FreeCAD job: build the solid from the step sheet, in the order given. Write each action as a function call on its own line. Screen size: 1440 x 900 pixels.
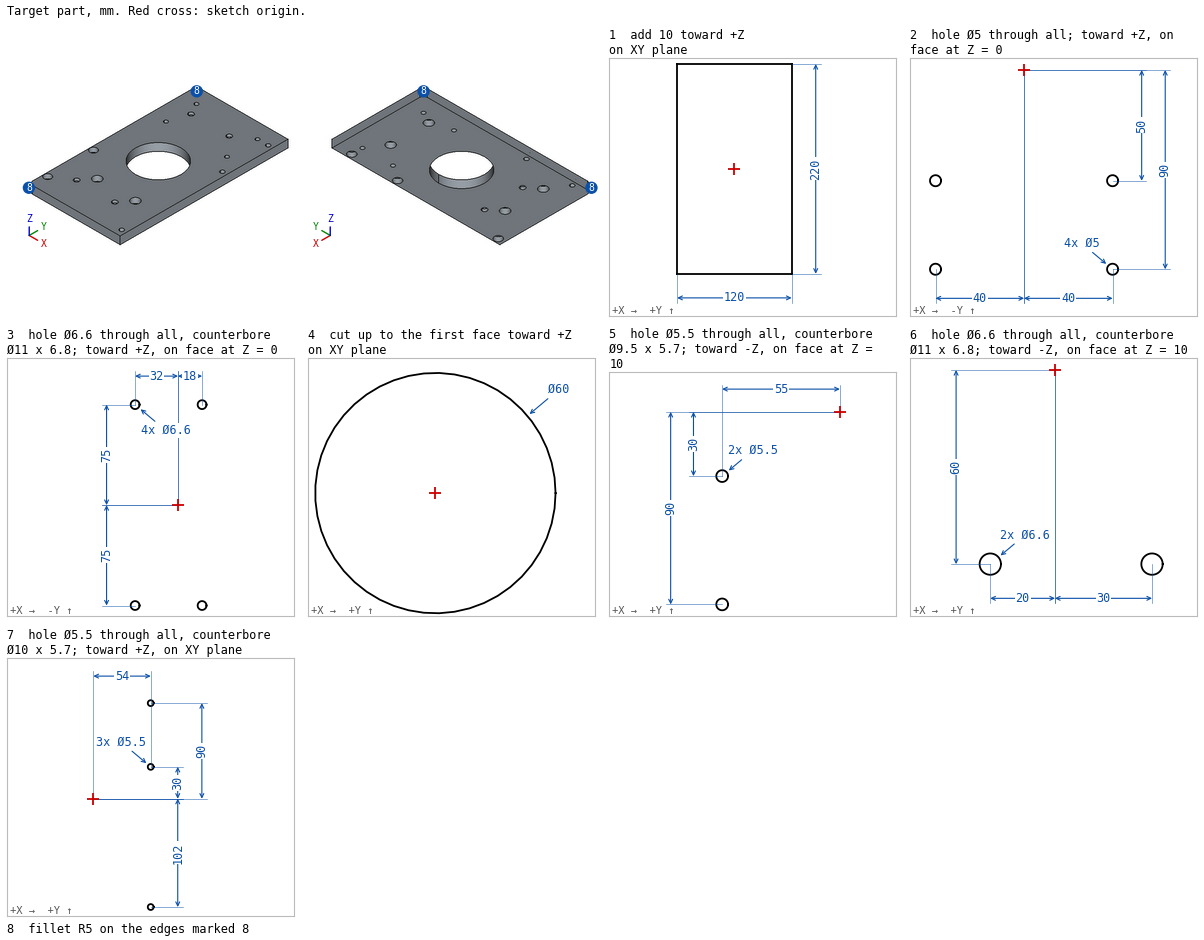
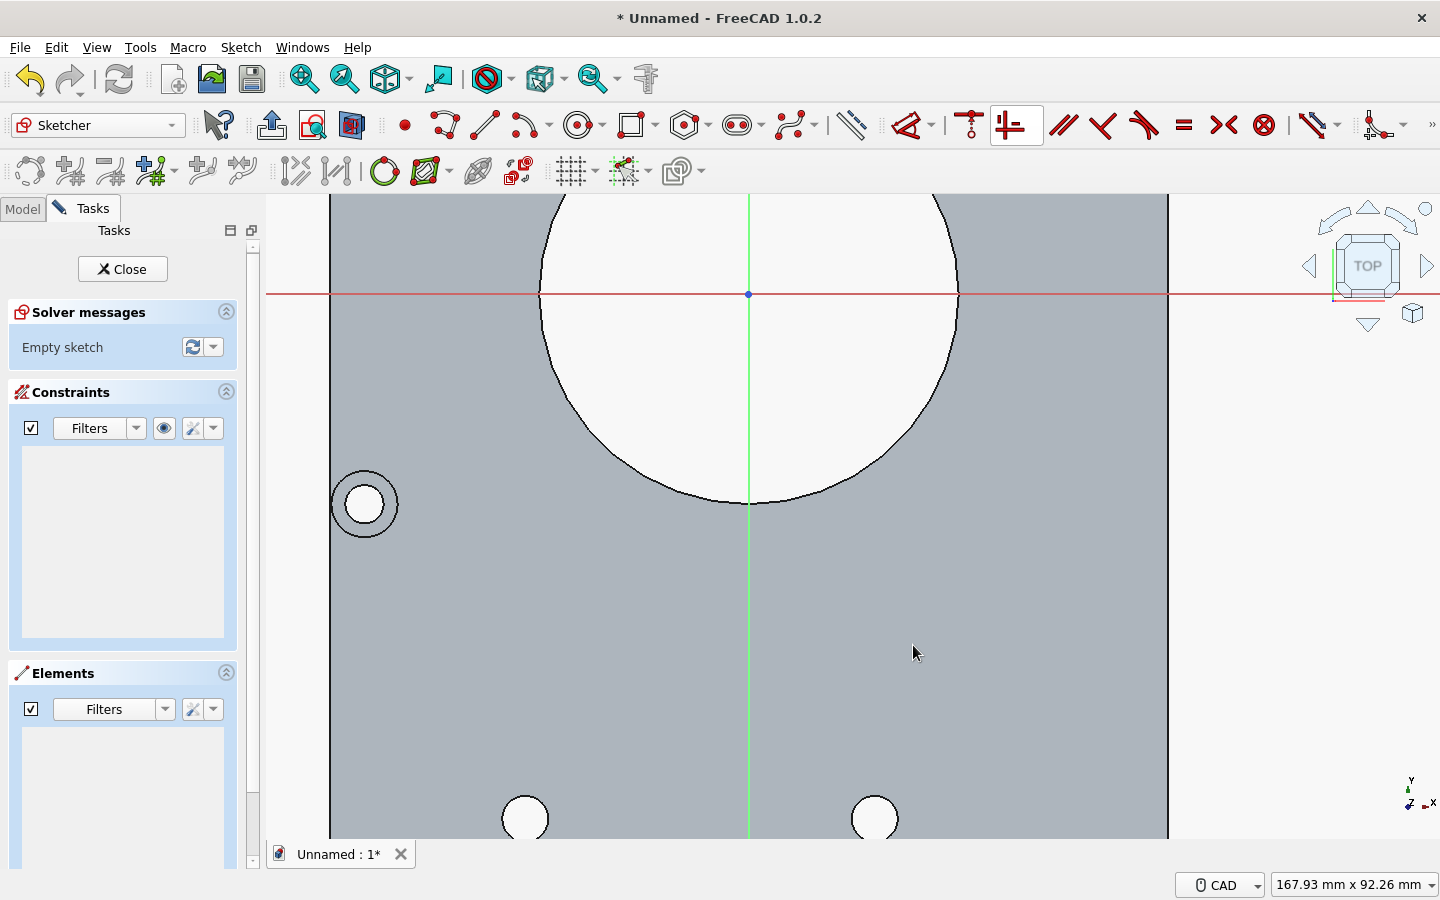
key(g)
key(c)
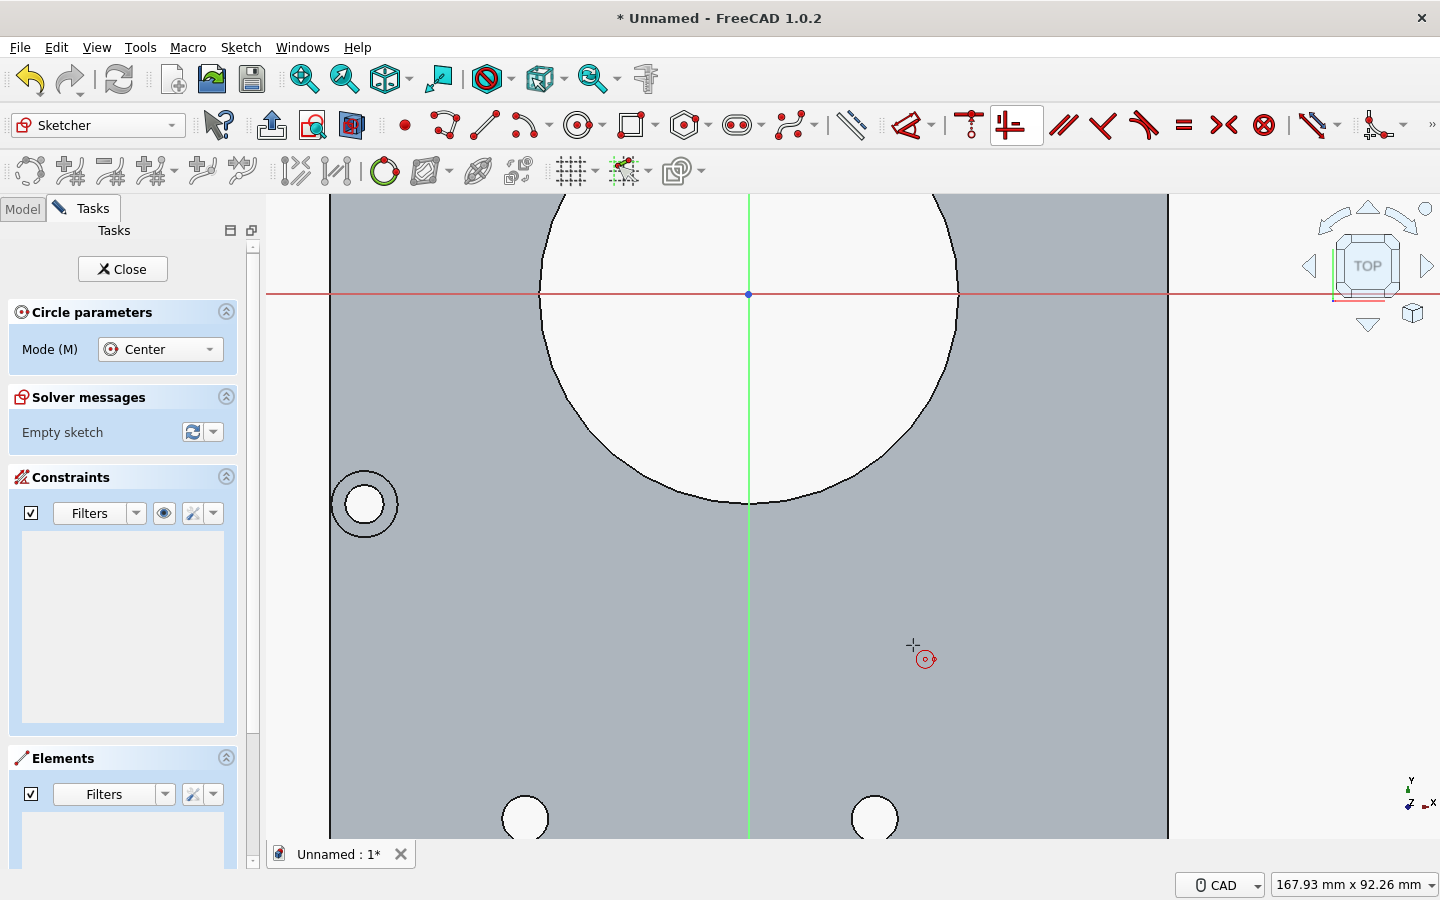
click(609, 714)
move(625, 698)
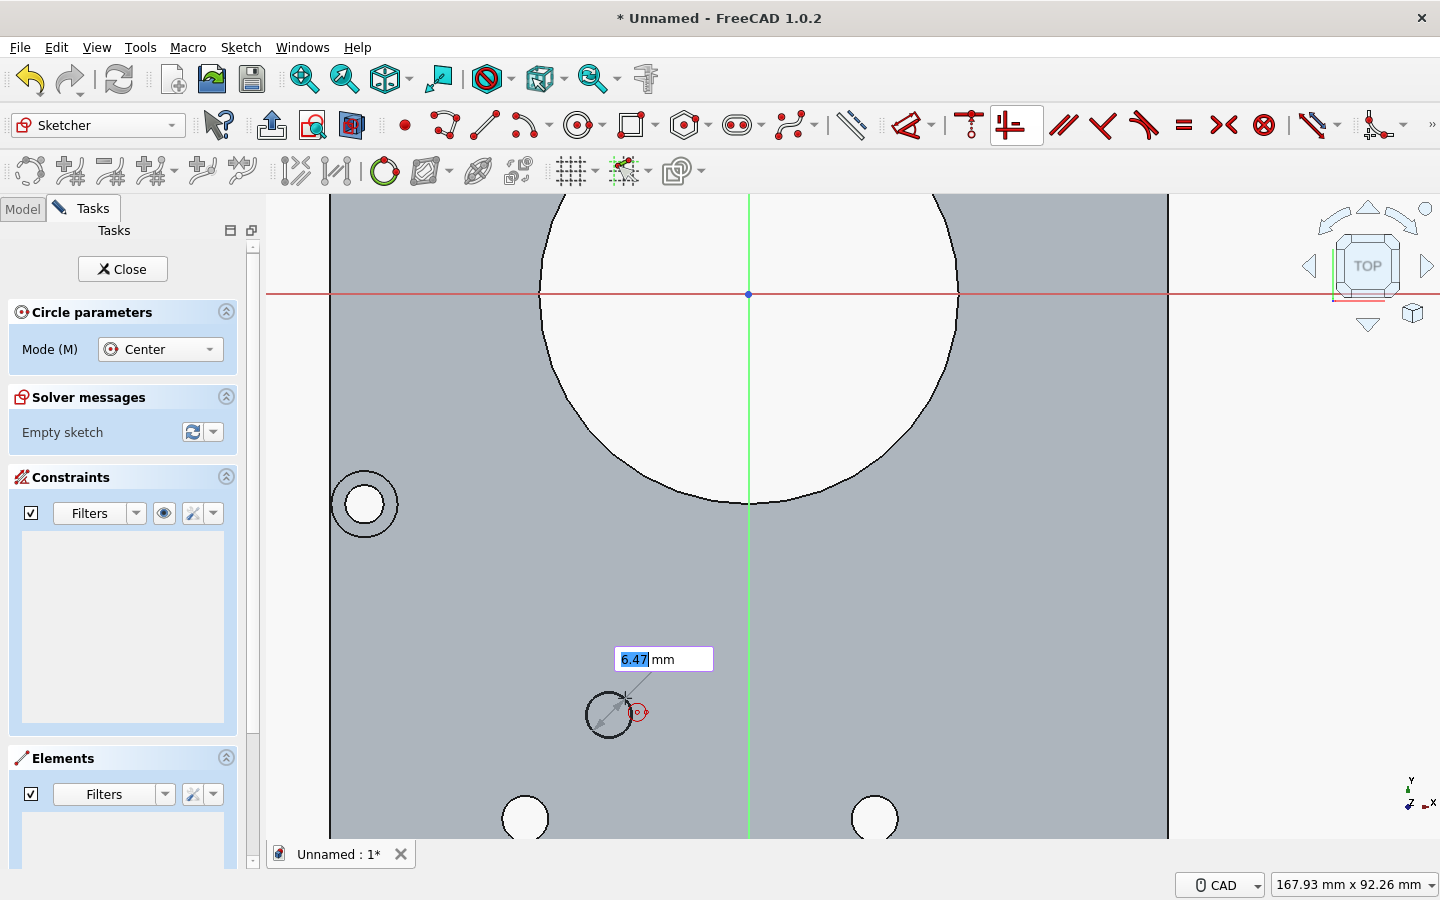
text(6.6)
key(Return)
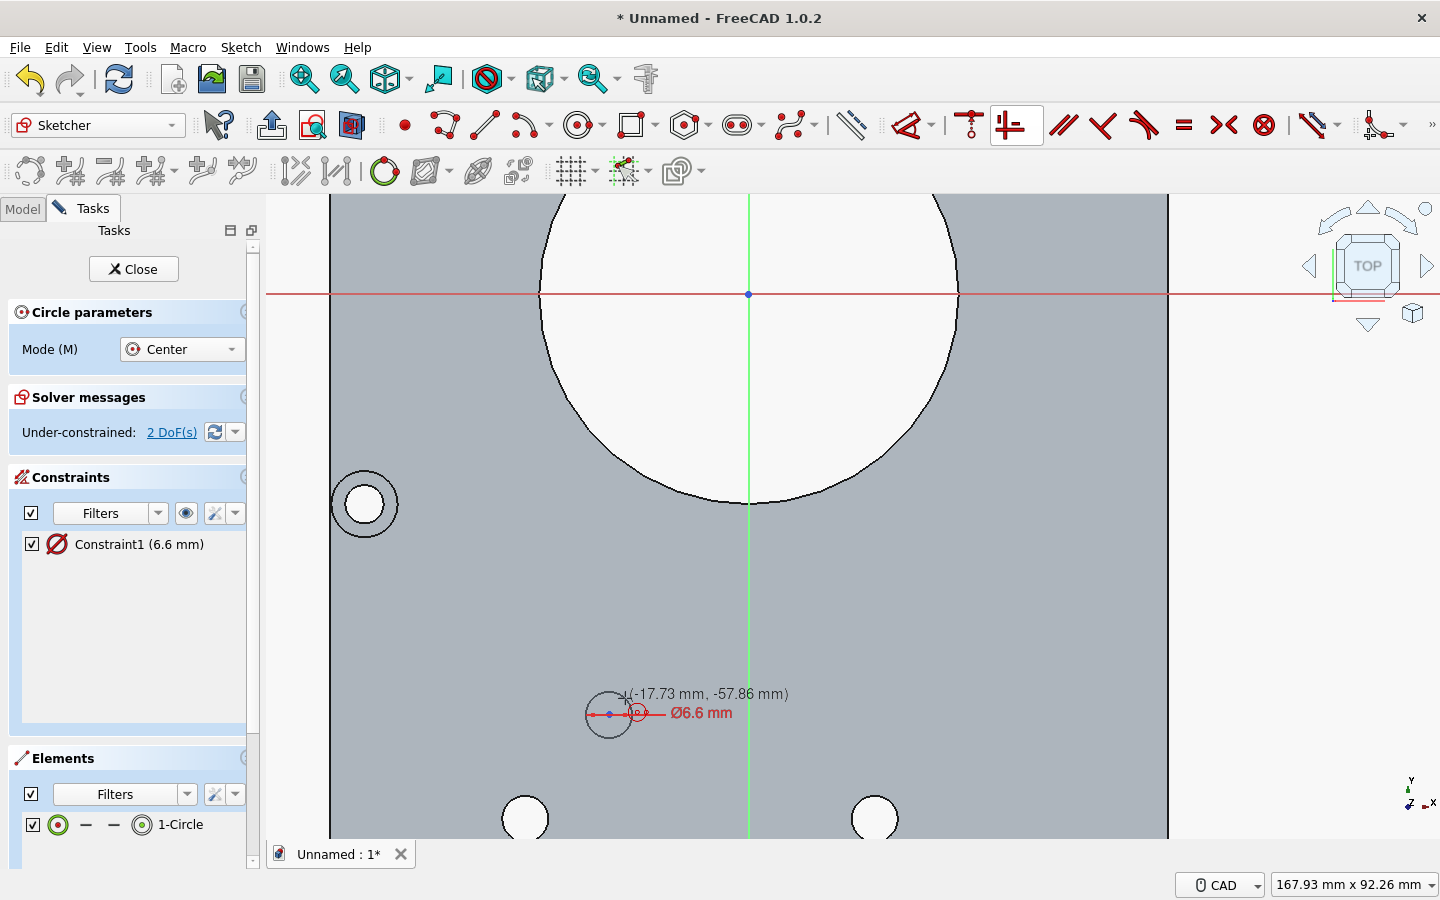
click(959, 714)
move(975, 698)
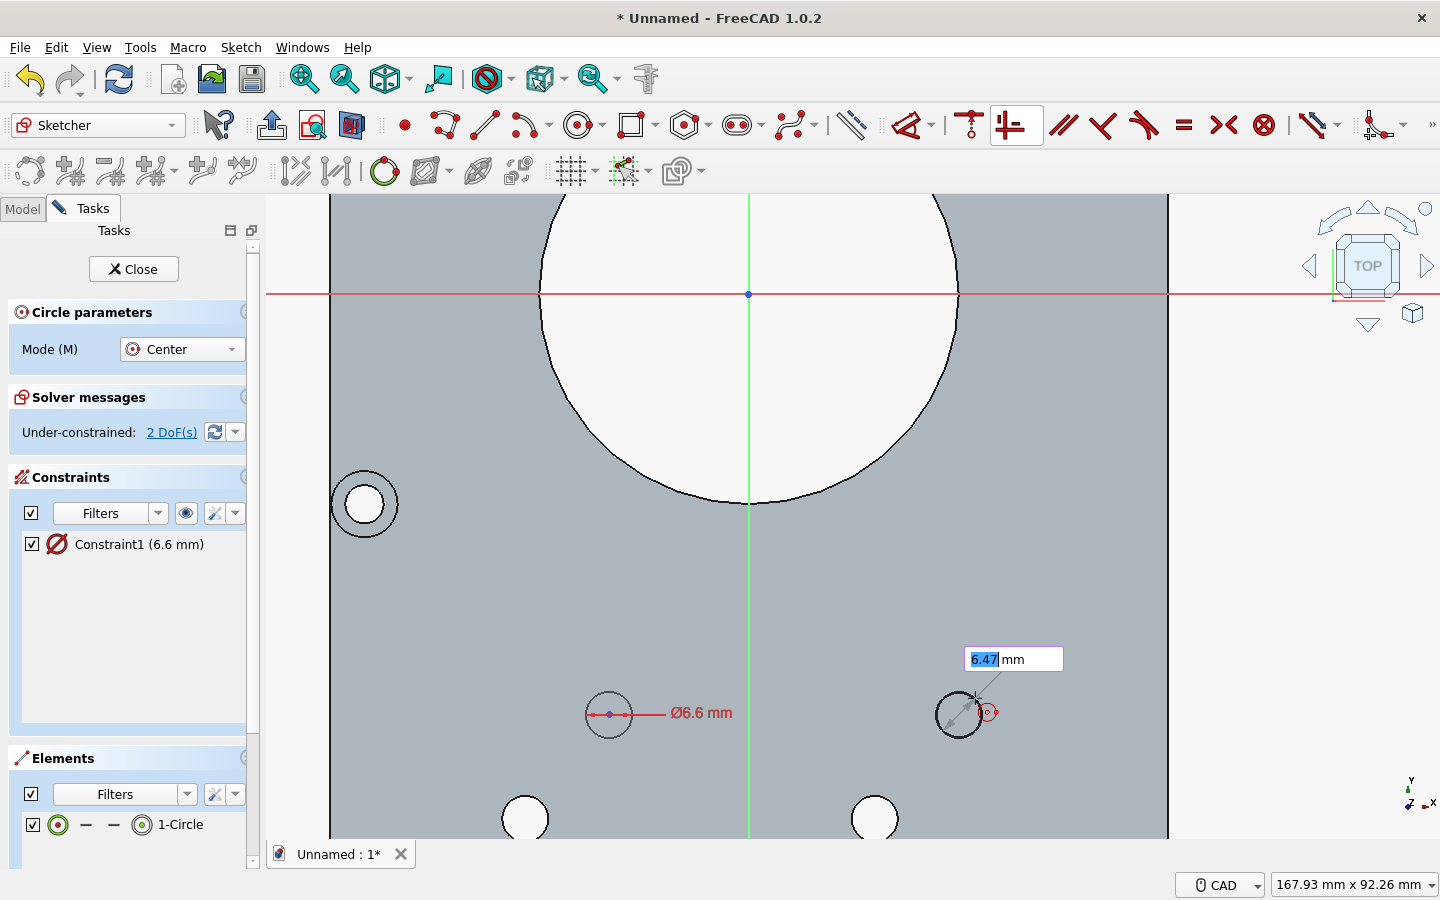
text(6.6)
key(Return)
key(Escape)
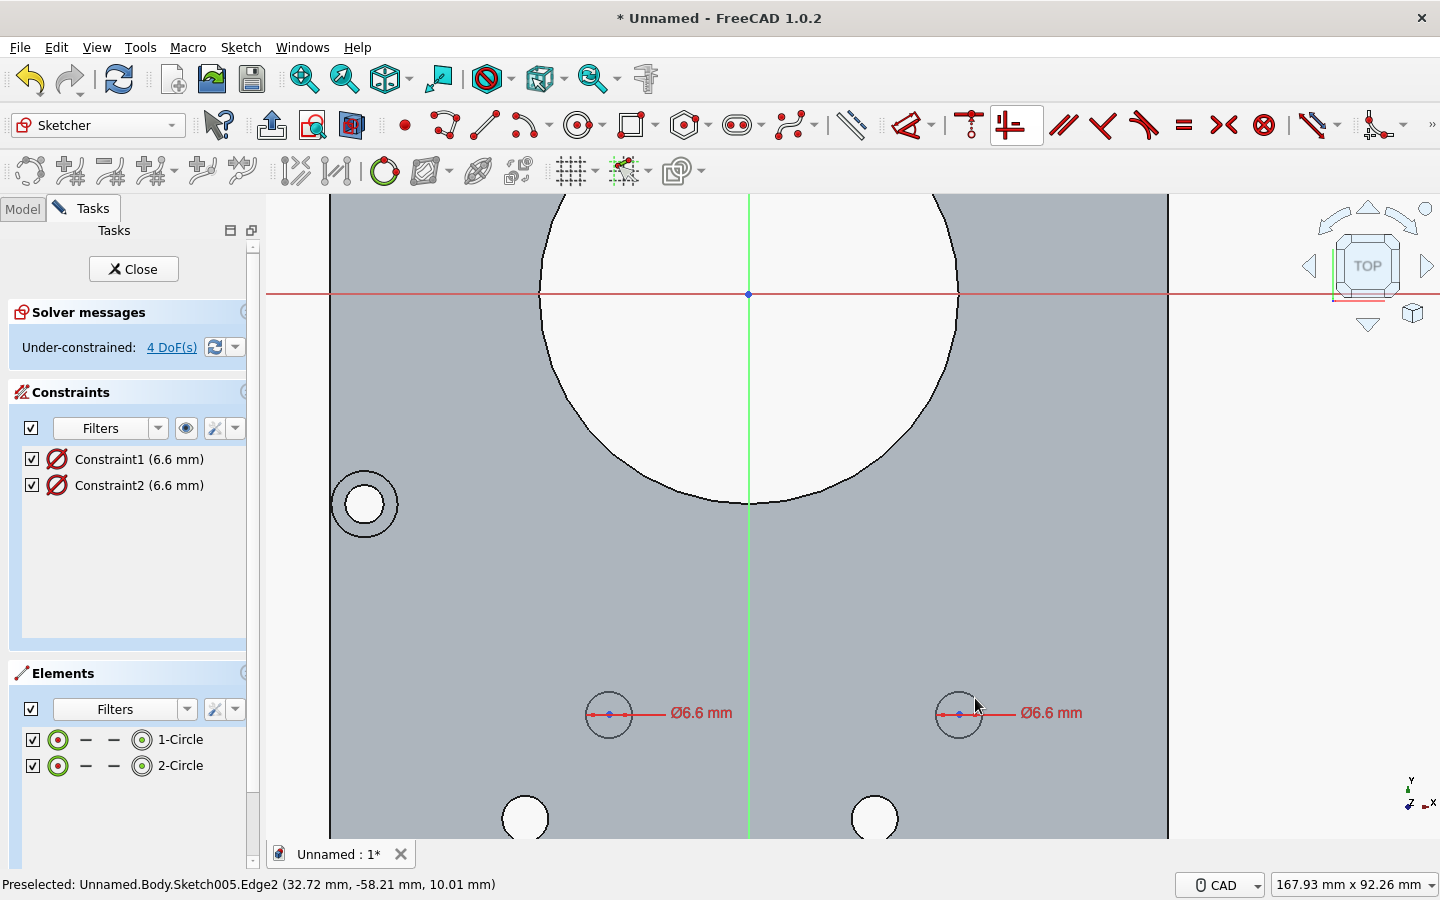
click(609, 715)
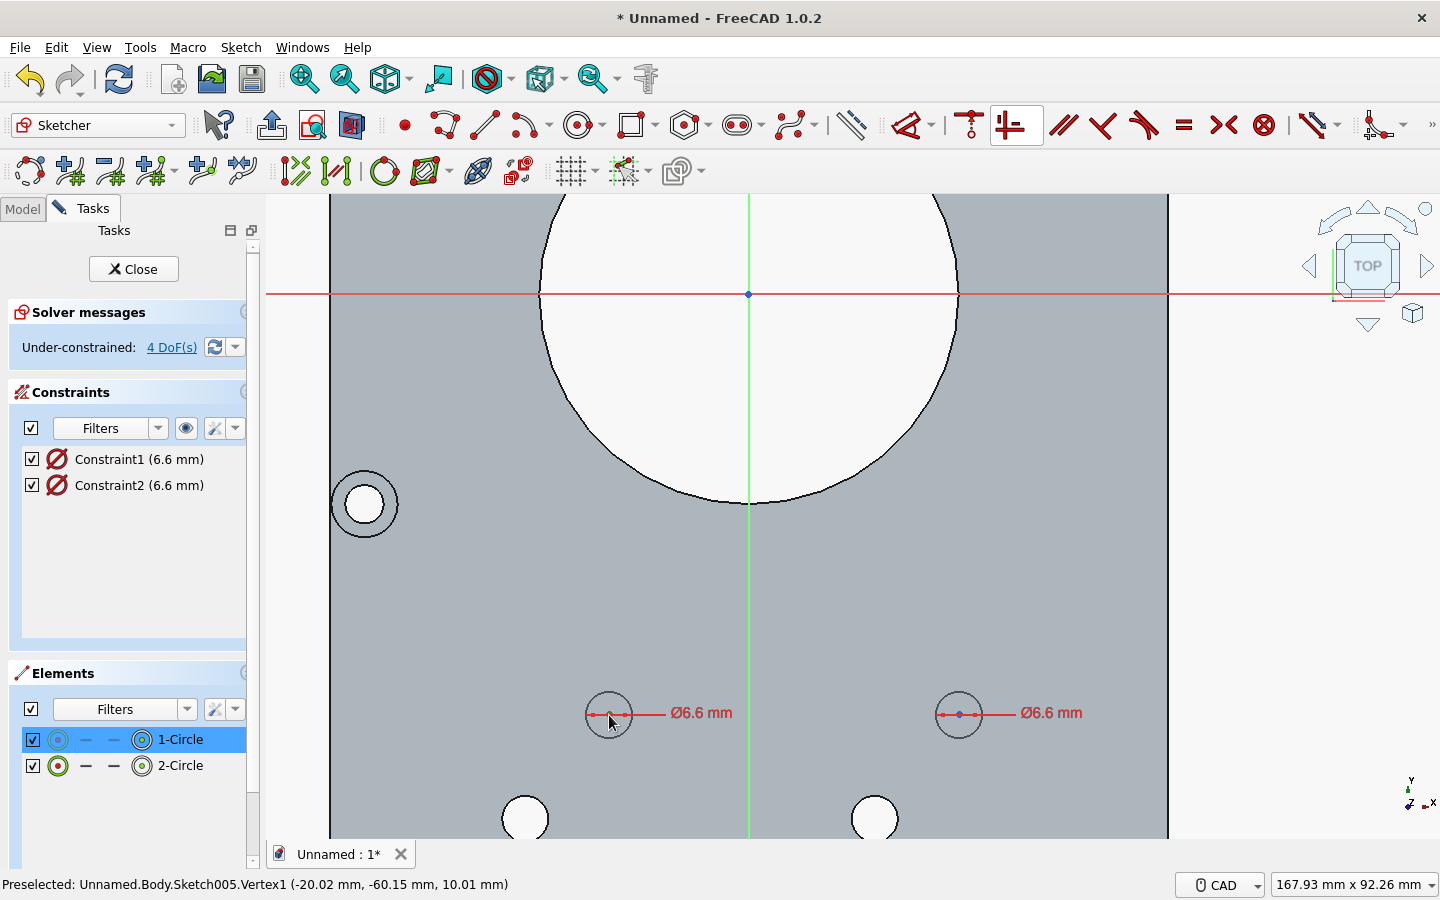
click(959, 715)